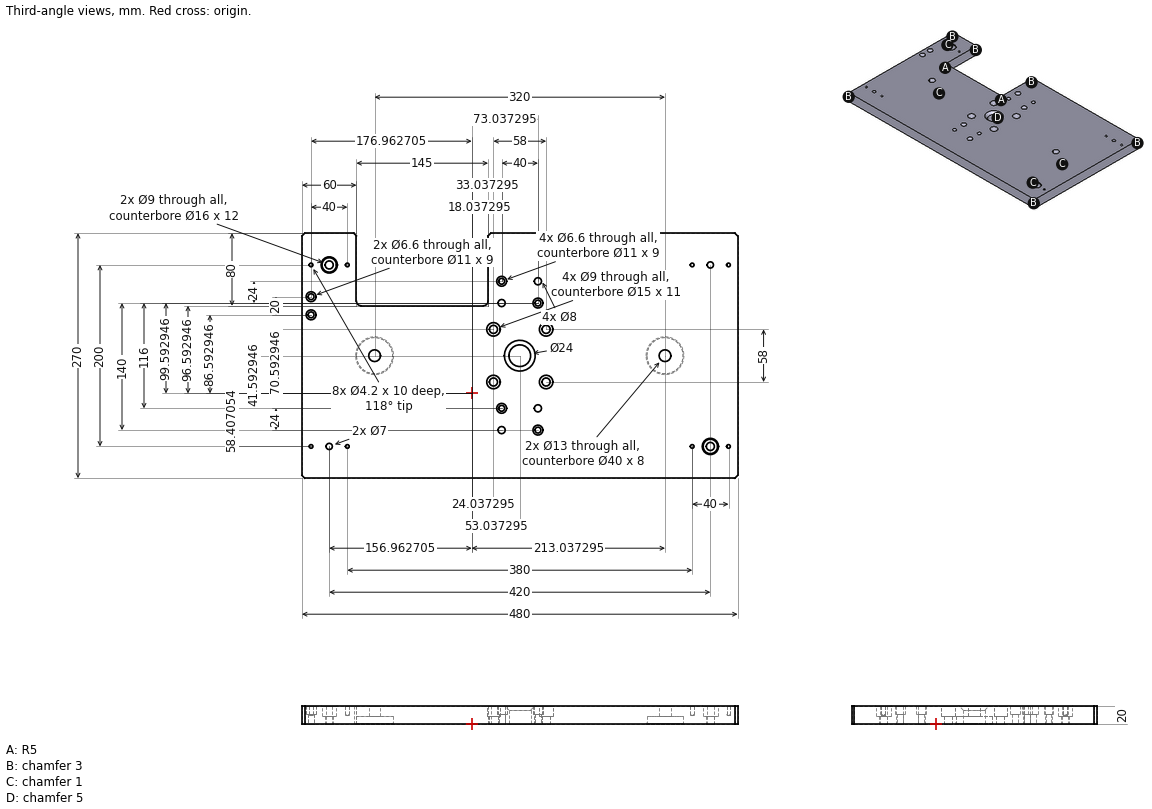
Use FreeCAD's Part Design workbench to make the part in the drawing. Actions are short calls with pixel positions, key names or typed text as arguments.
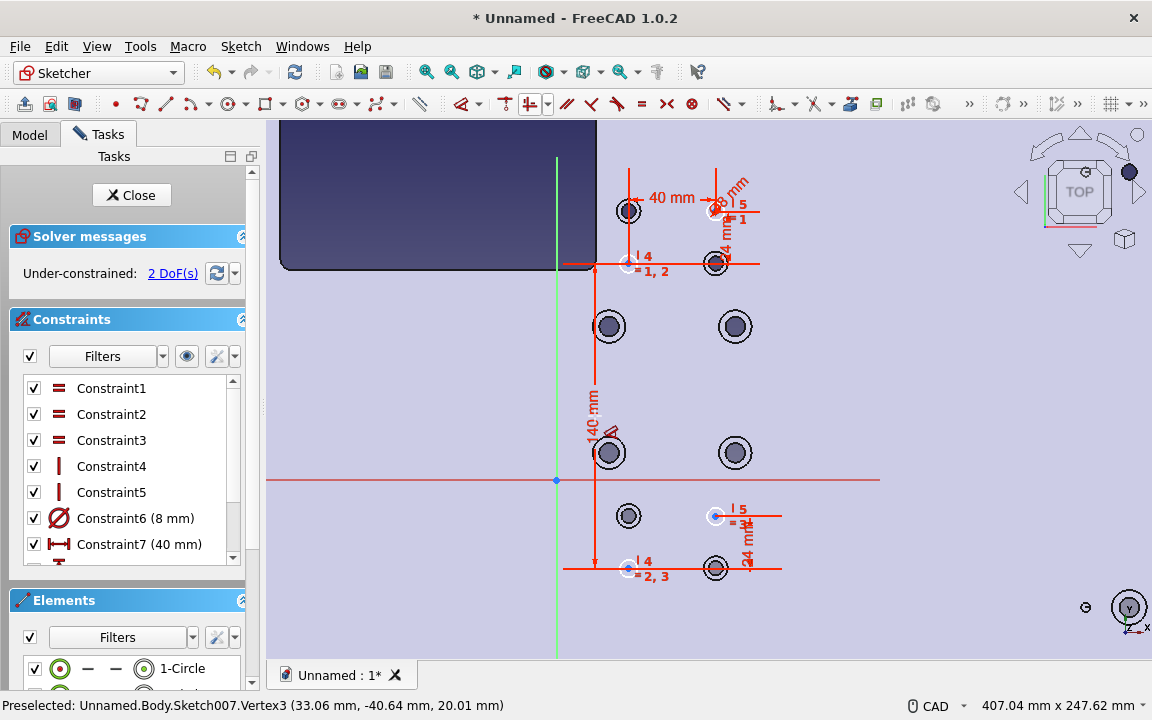
click(716, 212)
click(636, 178)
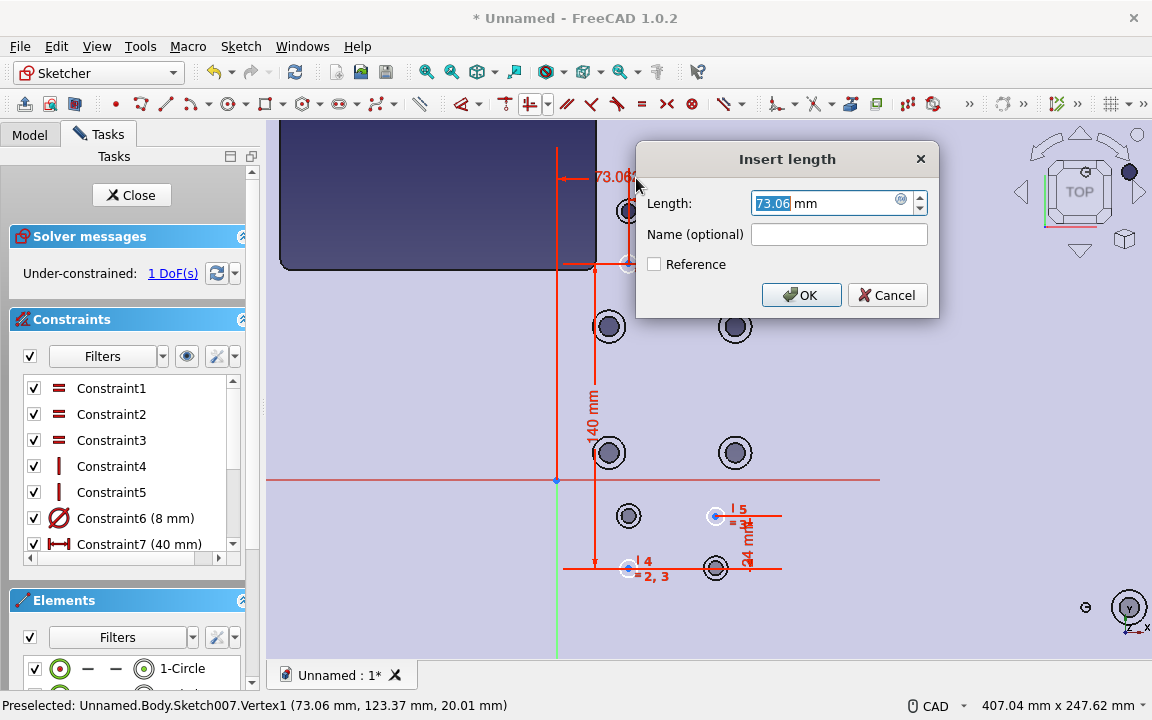
text(73.037295)
key(Return)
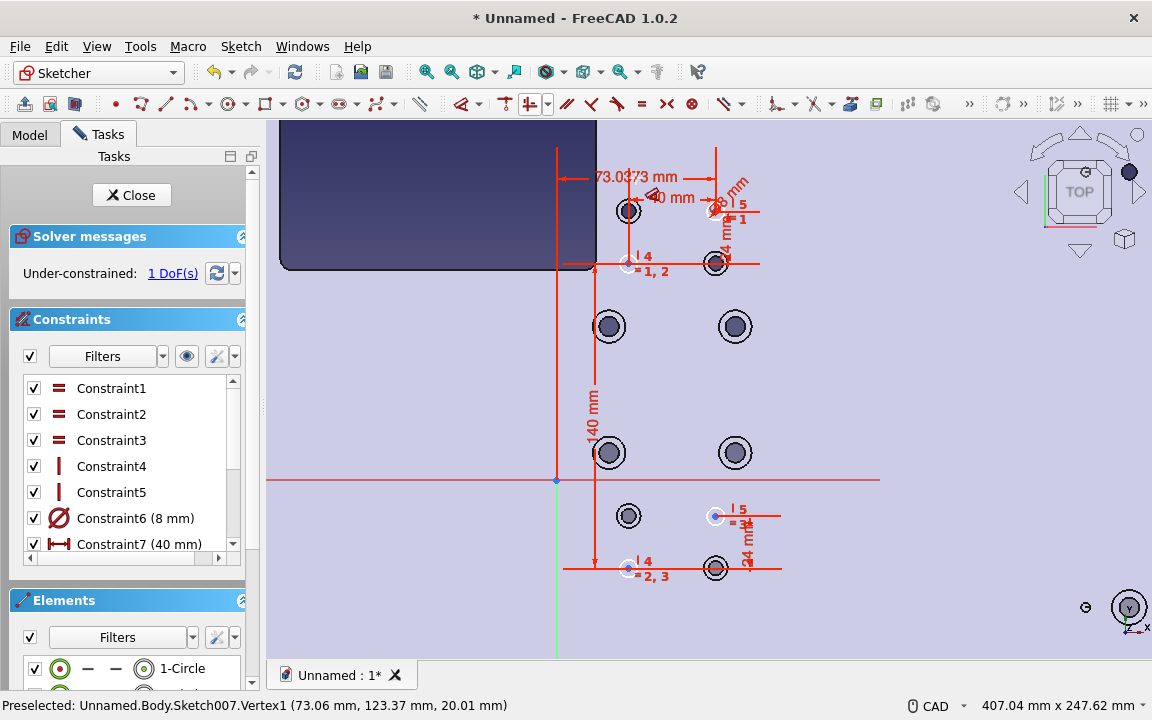
click(629, 264)
click(523, 372)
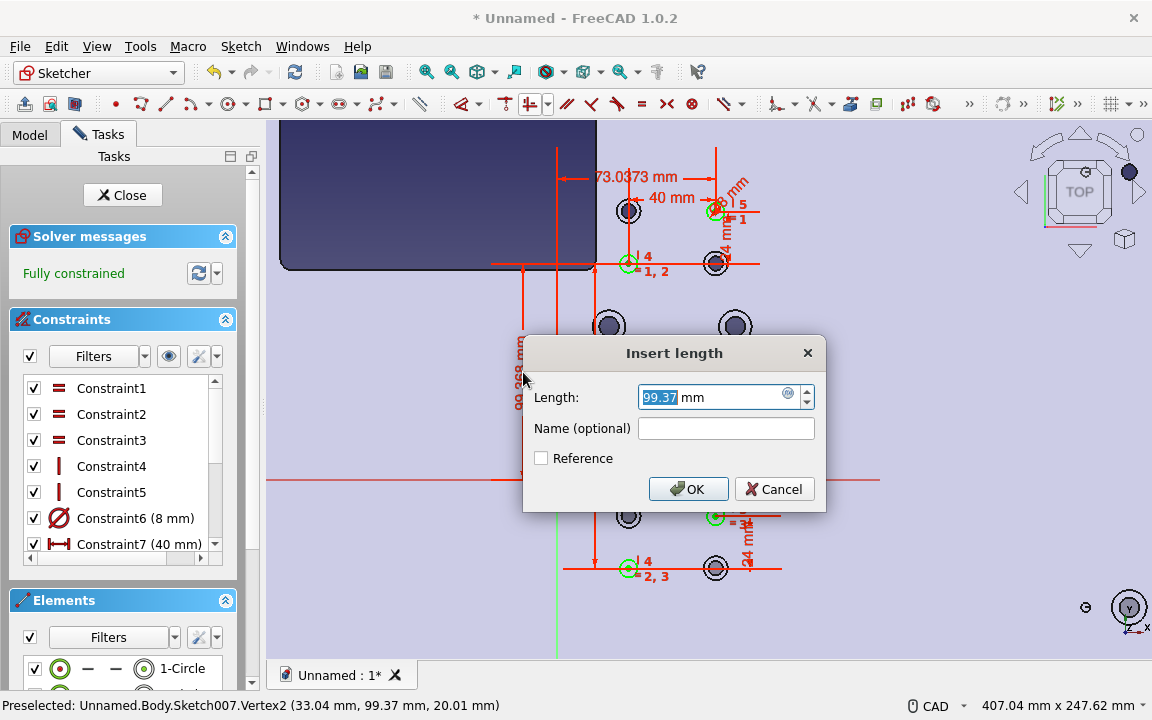
text(99.592946)
key(Return)
key(Escape)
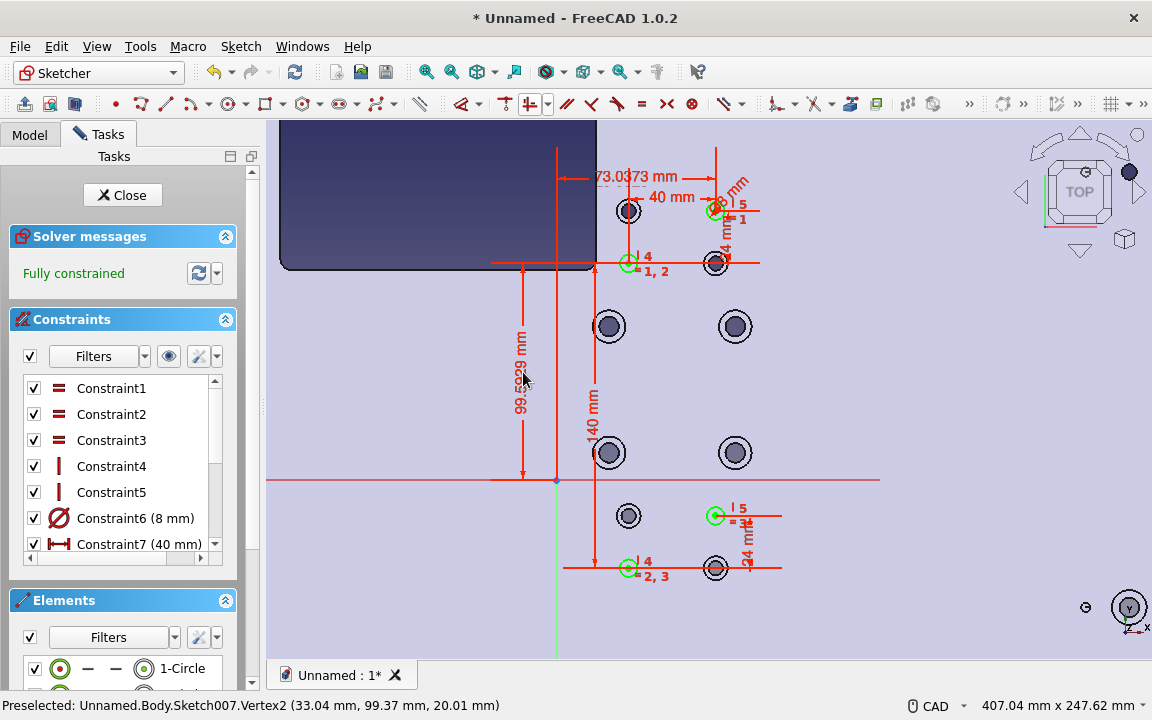
click(123, 195)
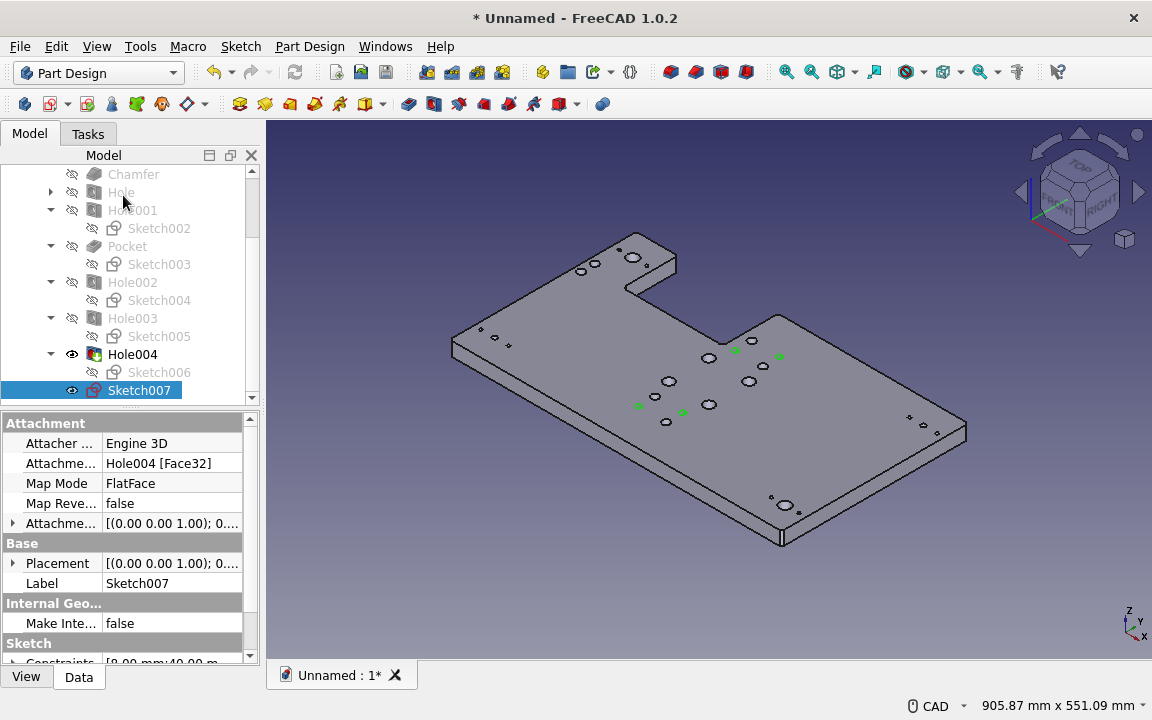
click(409, 104)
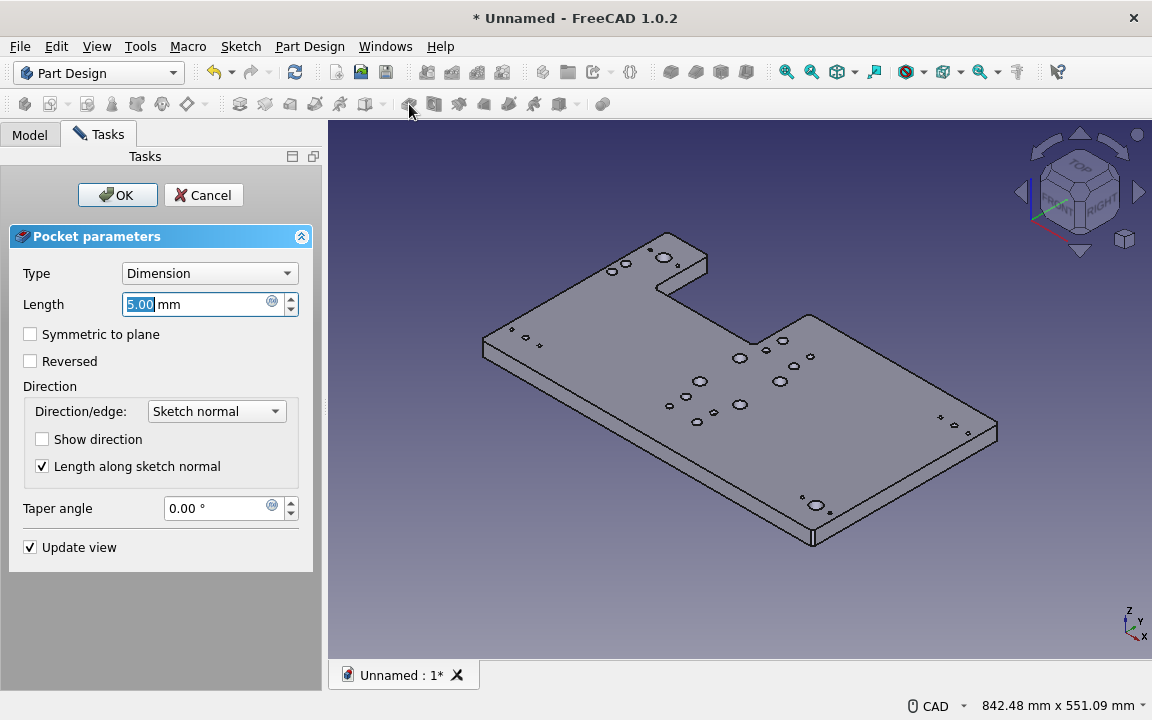
click(210, 274)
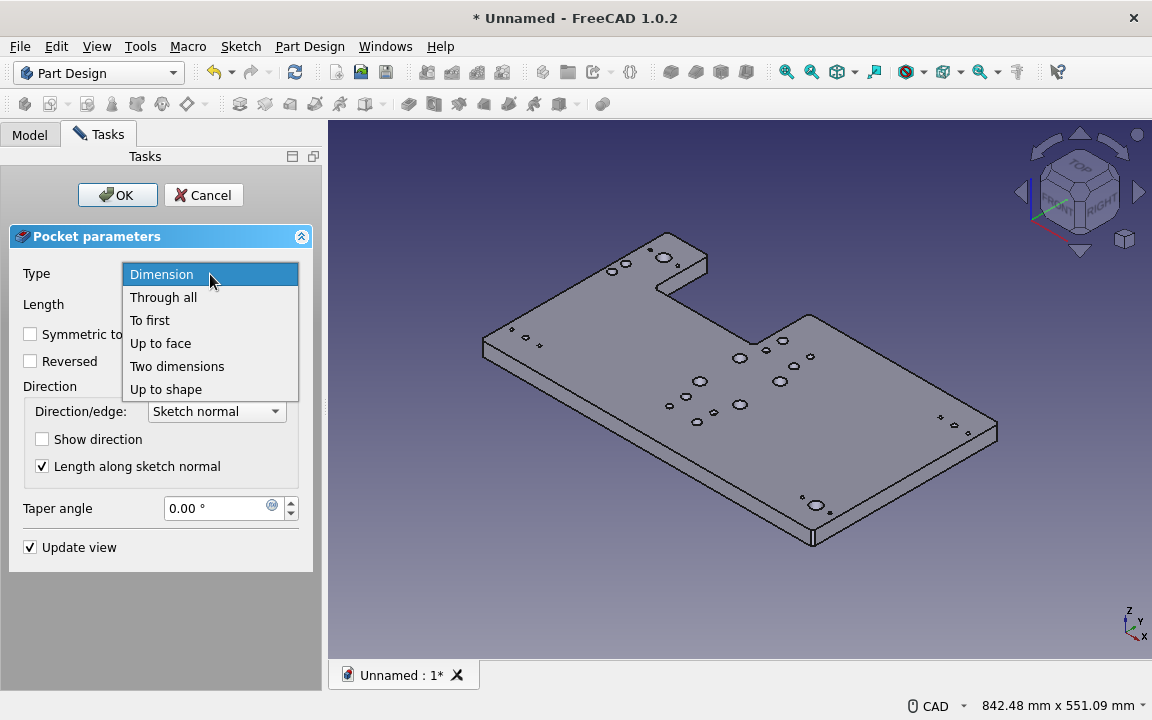
click(208, 298)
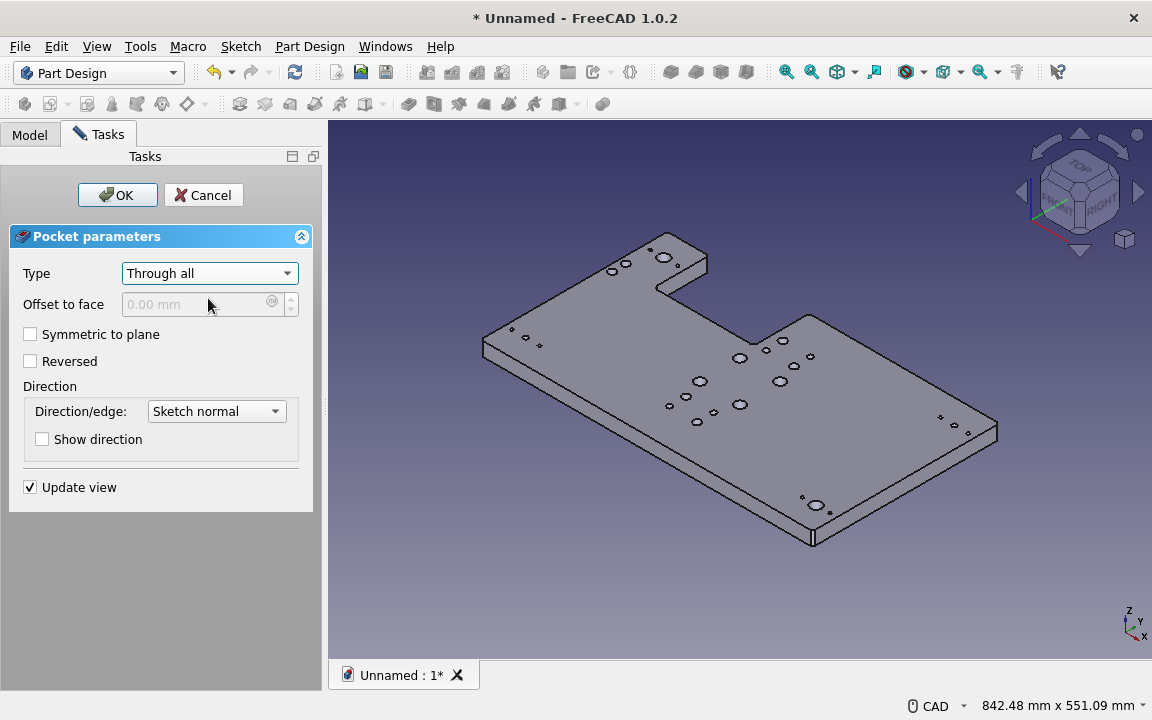
click(118, 195)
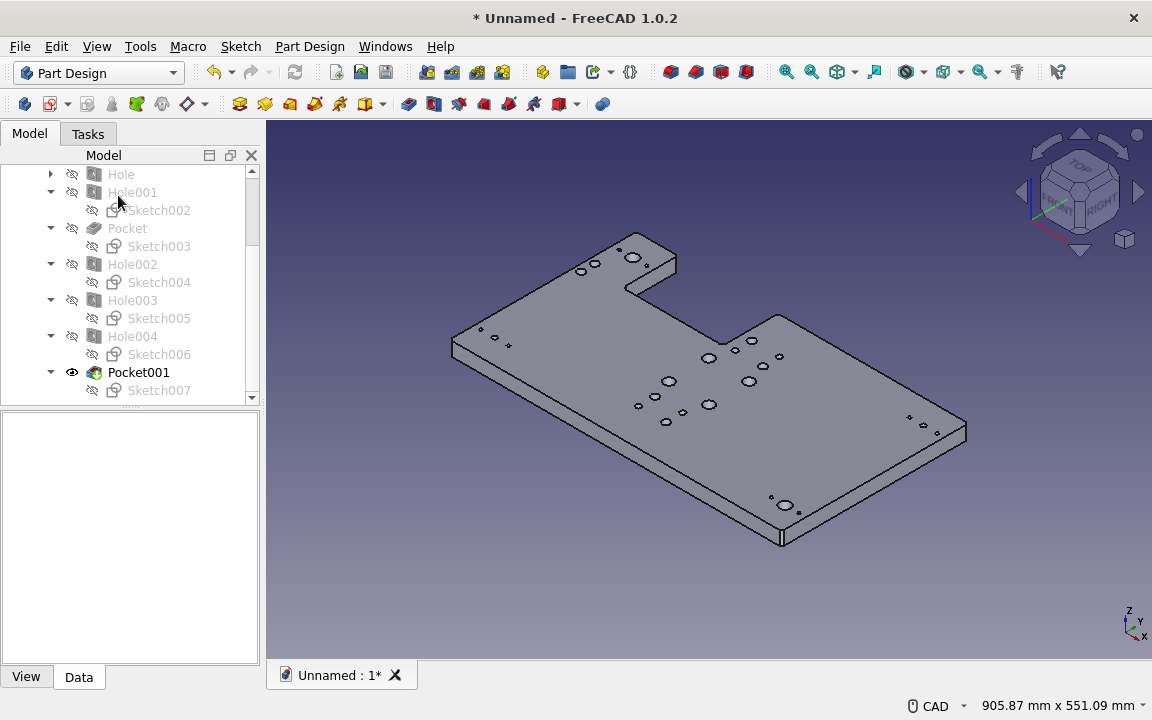
click(804, 435)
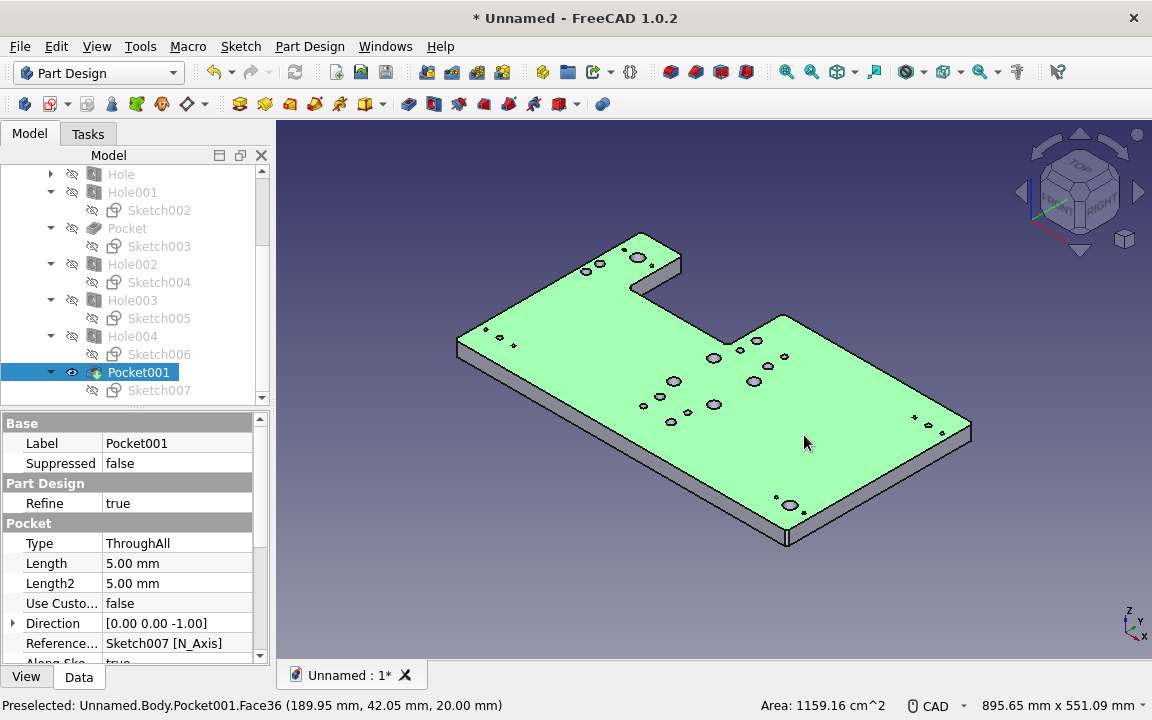
click(50, 104)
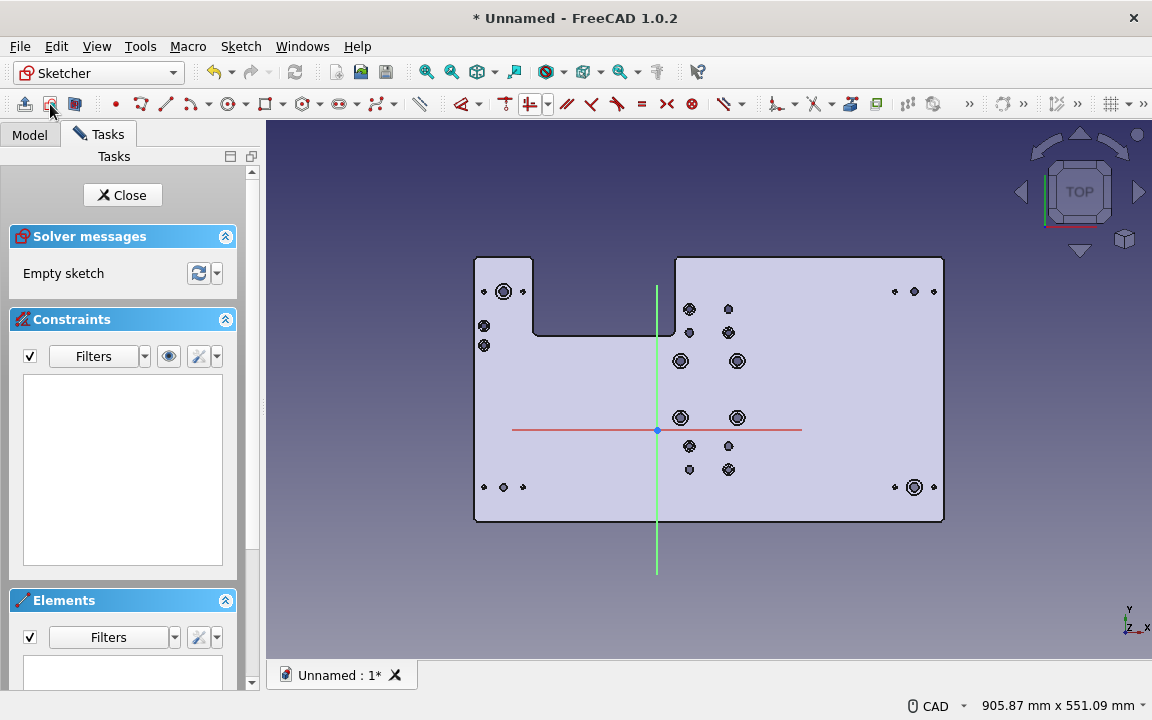
scroll(714, 390, up, 13)